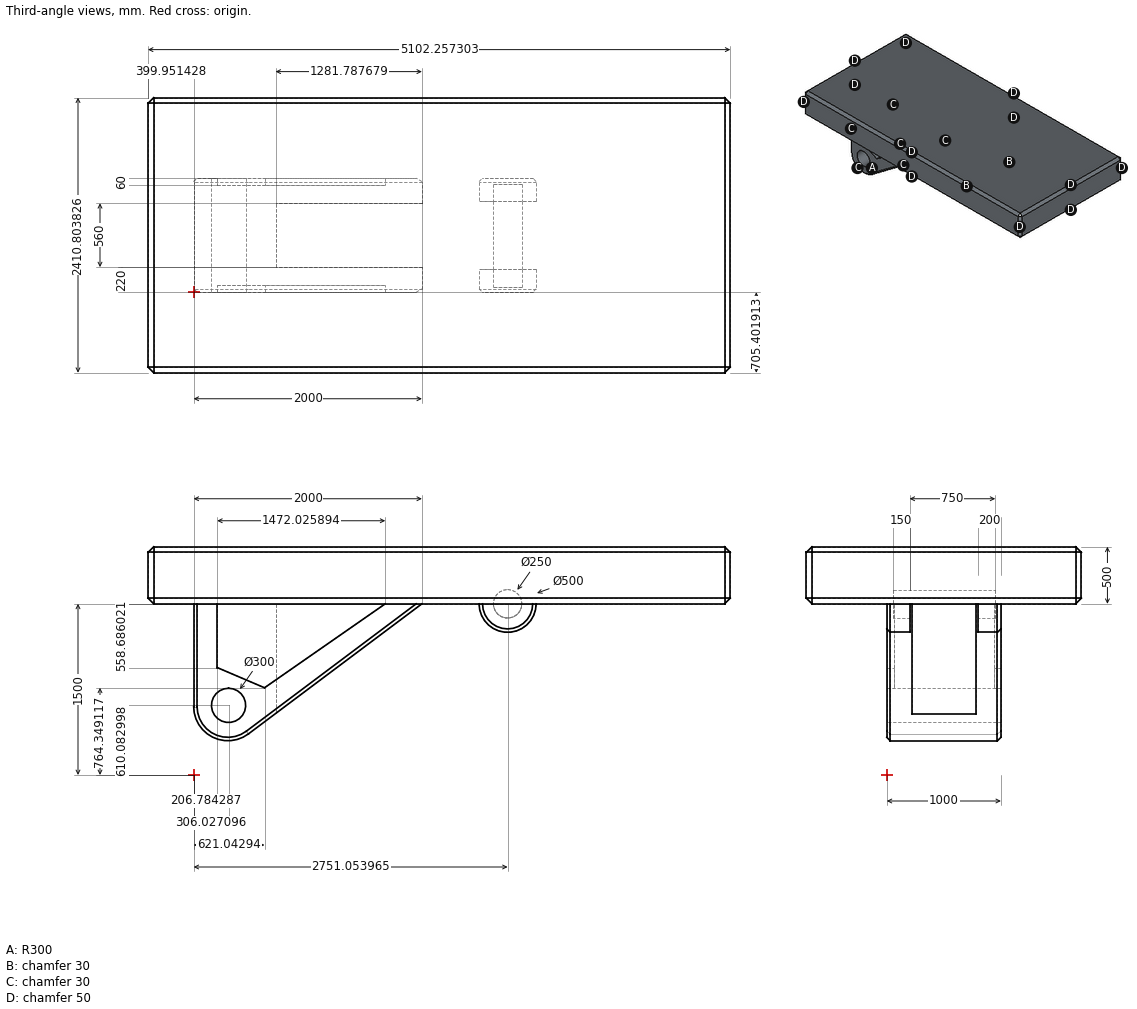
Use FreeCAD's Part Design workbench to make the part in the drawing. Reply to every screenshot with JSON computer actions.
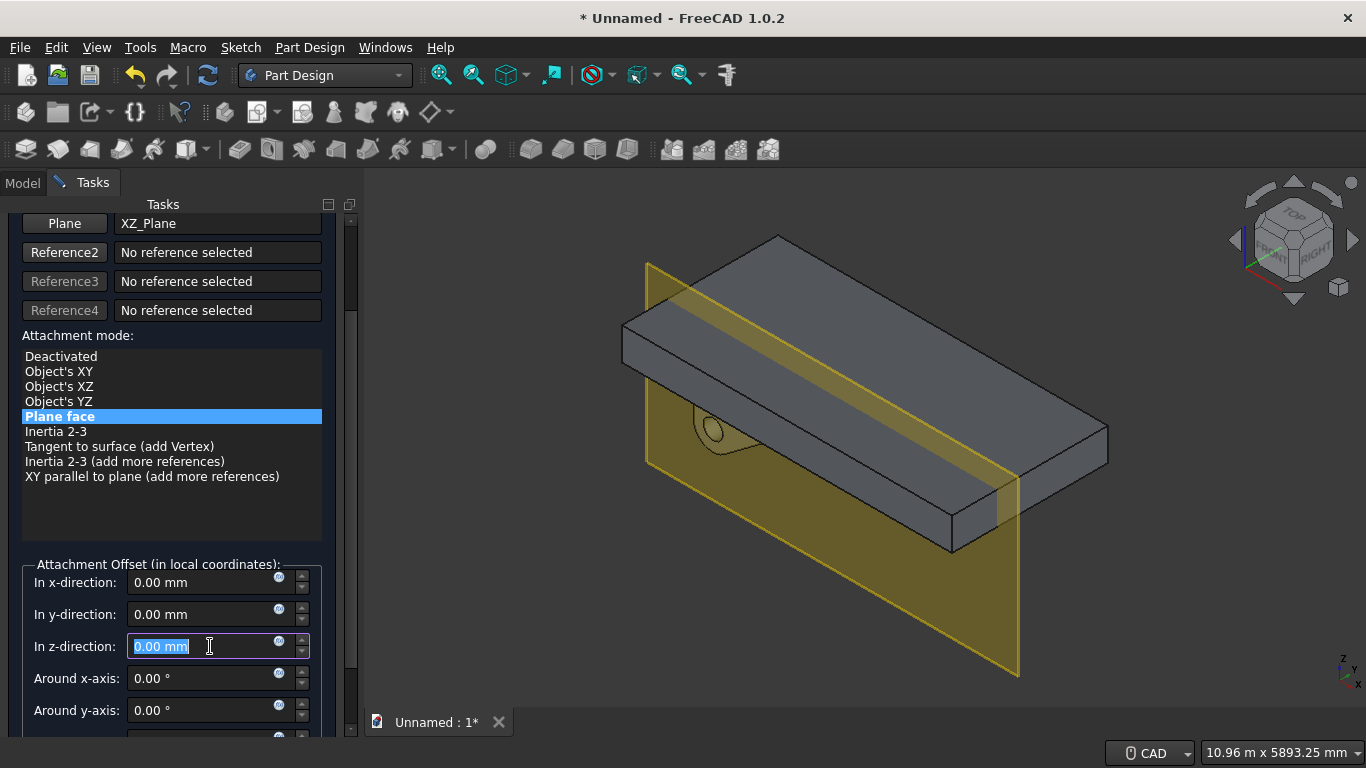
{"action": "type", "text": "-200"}
{"action": "key", "text": "Tab"}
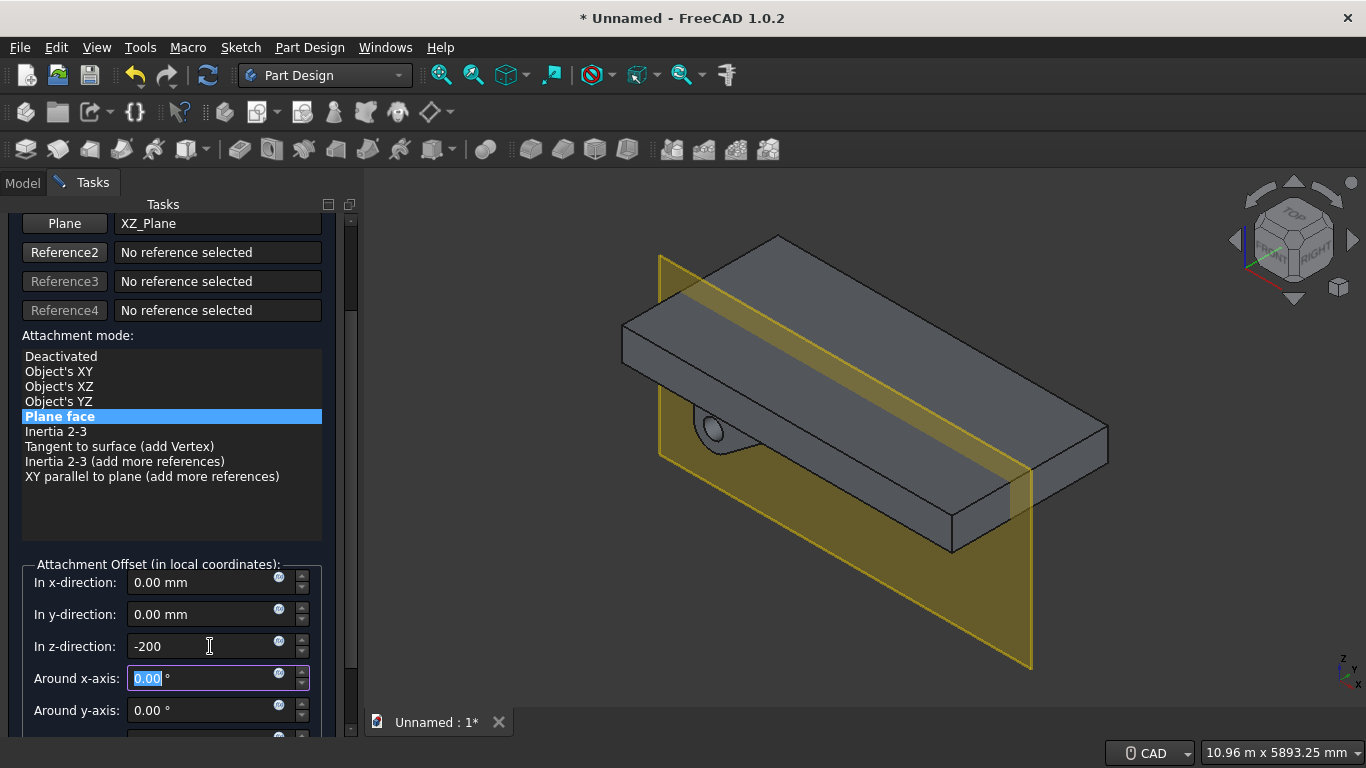
{"action": "scroll", "coordinate": [351, 475], "scroll_direction": "up", "scroll_amount": 3}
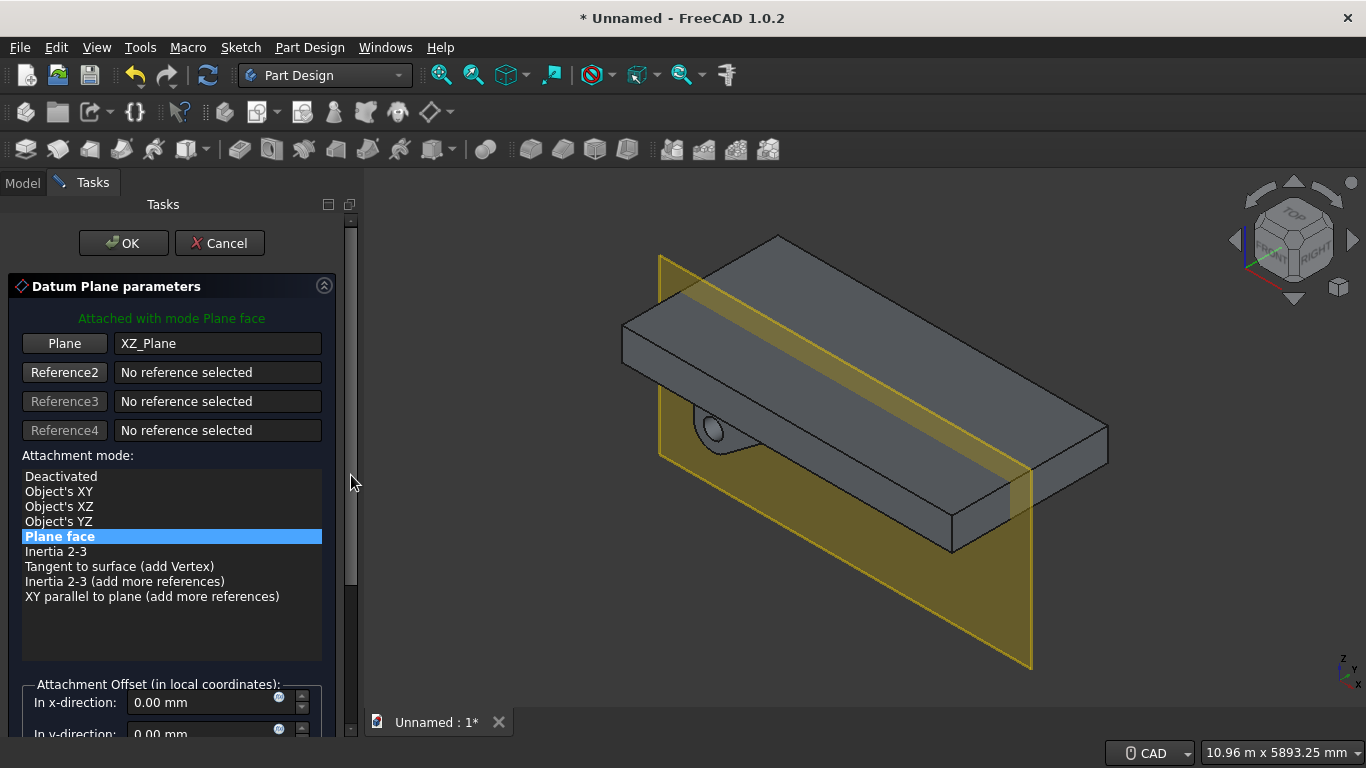
{"action": "left_click", "coordinate": [124, 243]}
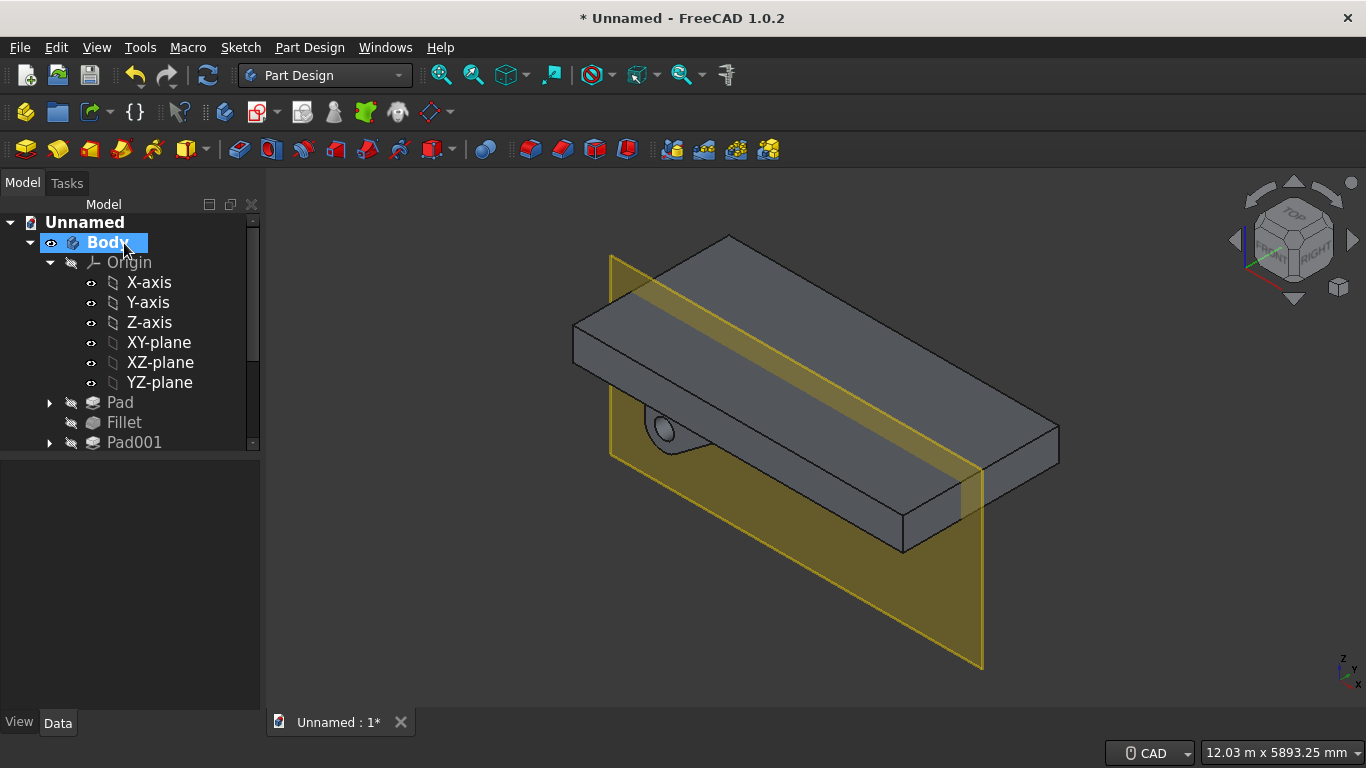
{"action": "scroll", "coordinate": [100, 338], "scroll_direction": "down", "scroll_amount": 3}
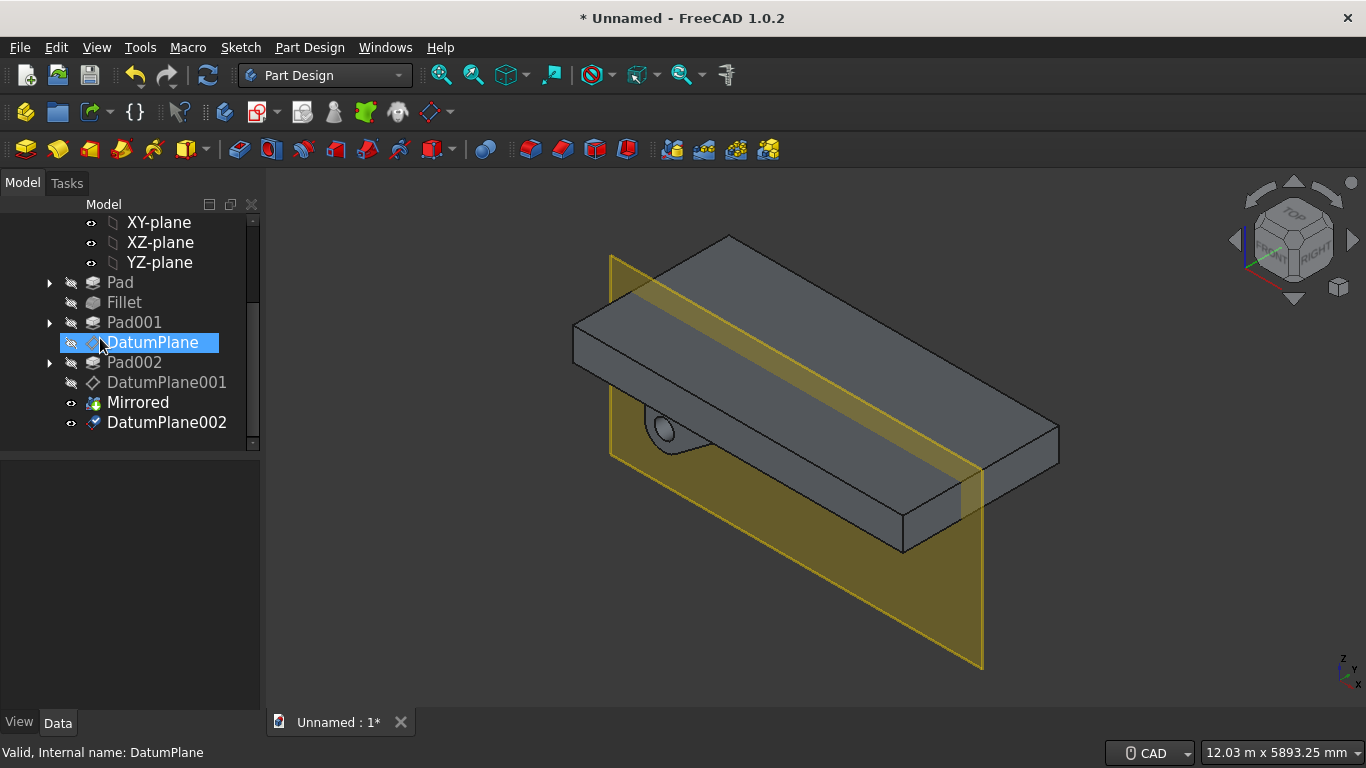
{"action": "left_click", "coordinate": [116, 423]}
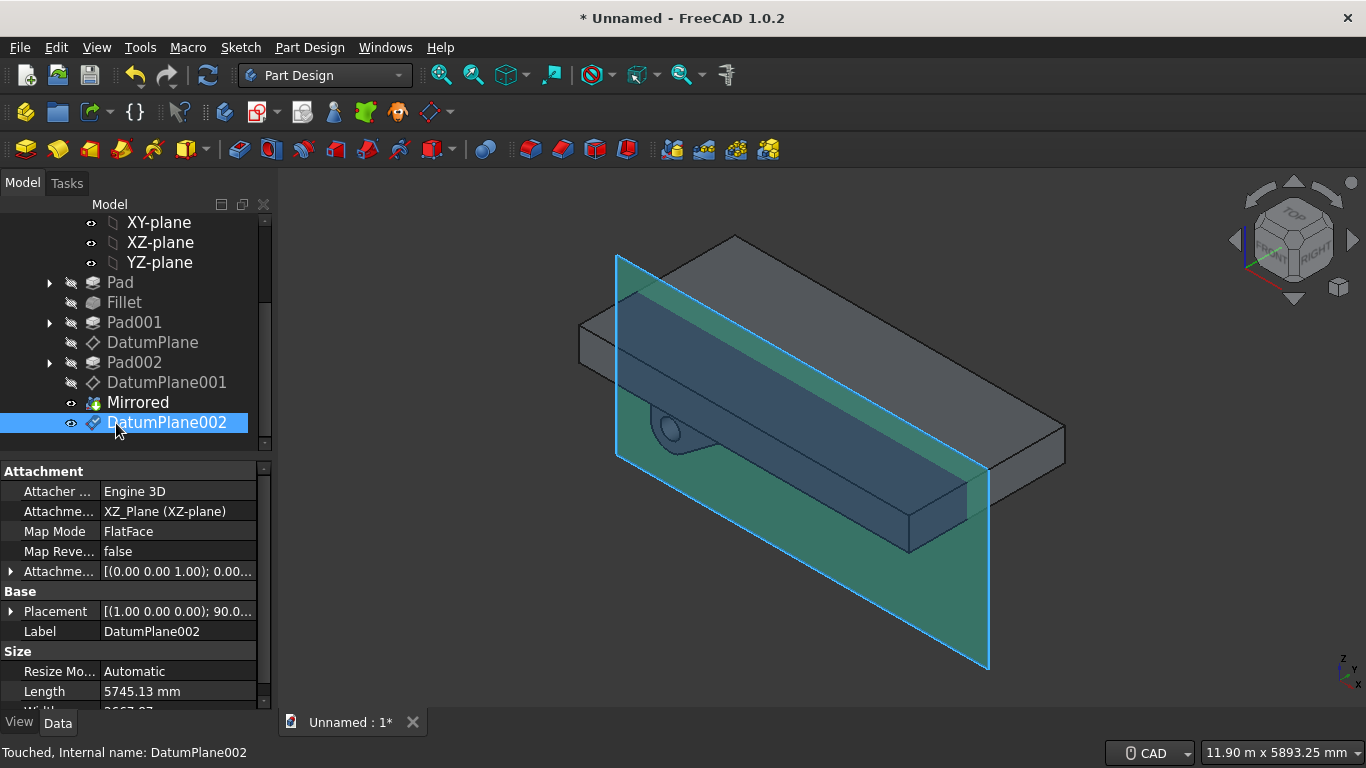
{"action": "left_click", "coordinate": [258, 112]}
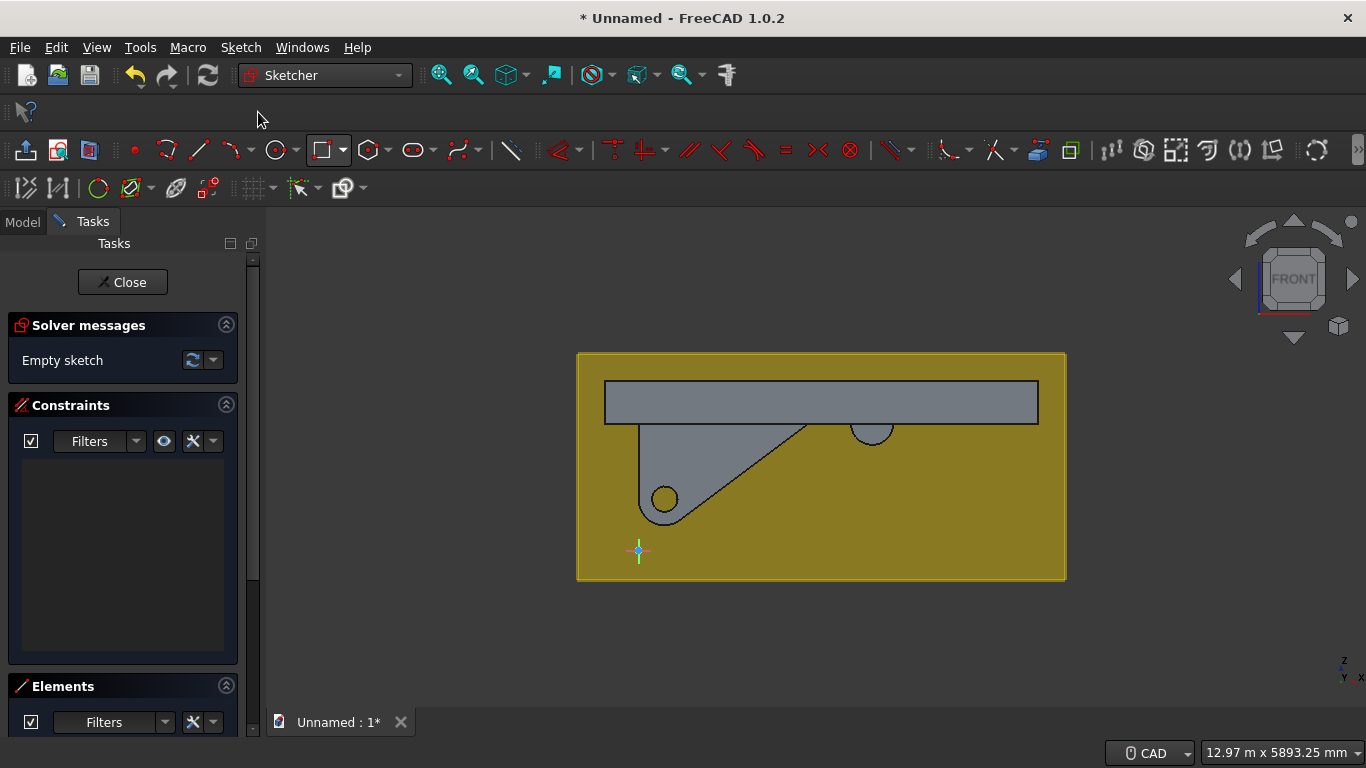
{"action": "key", "text": "q s"}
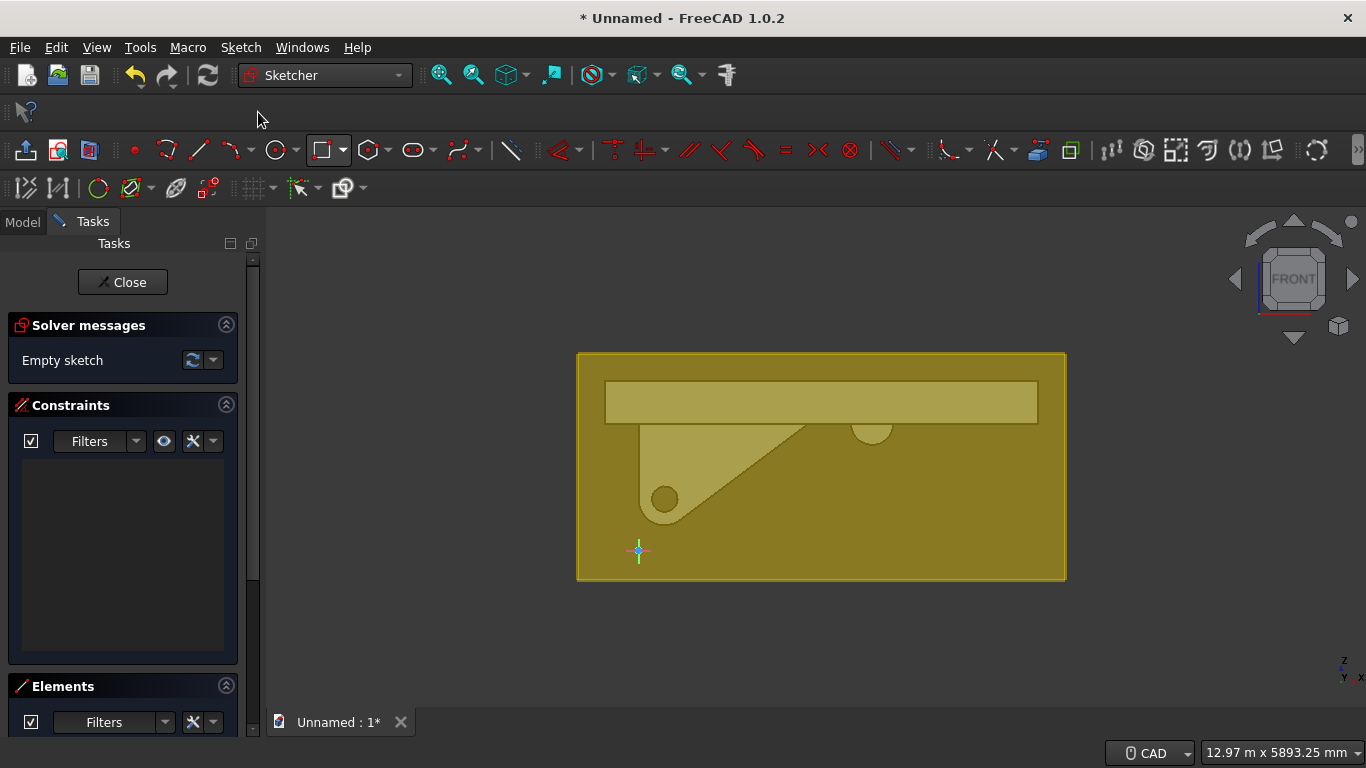
{"action": "scroll", "coordinate": [882, 421], "scroll_direction": "up", "scroll_amount": 13}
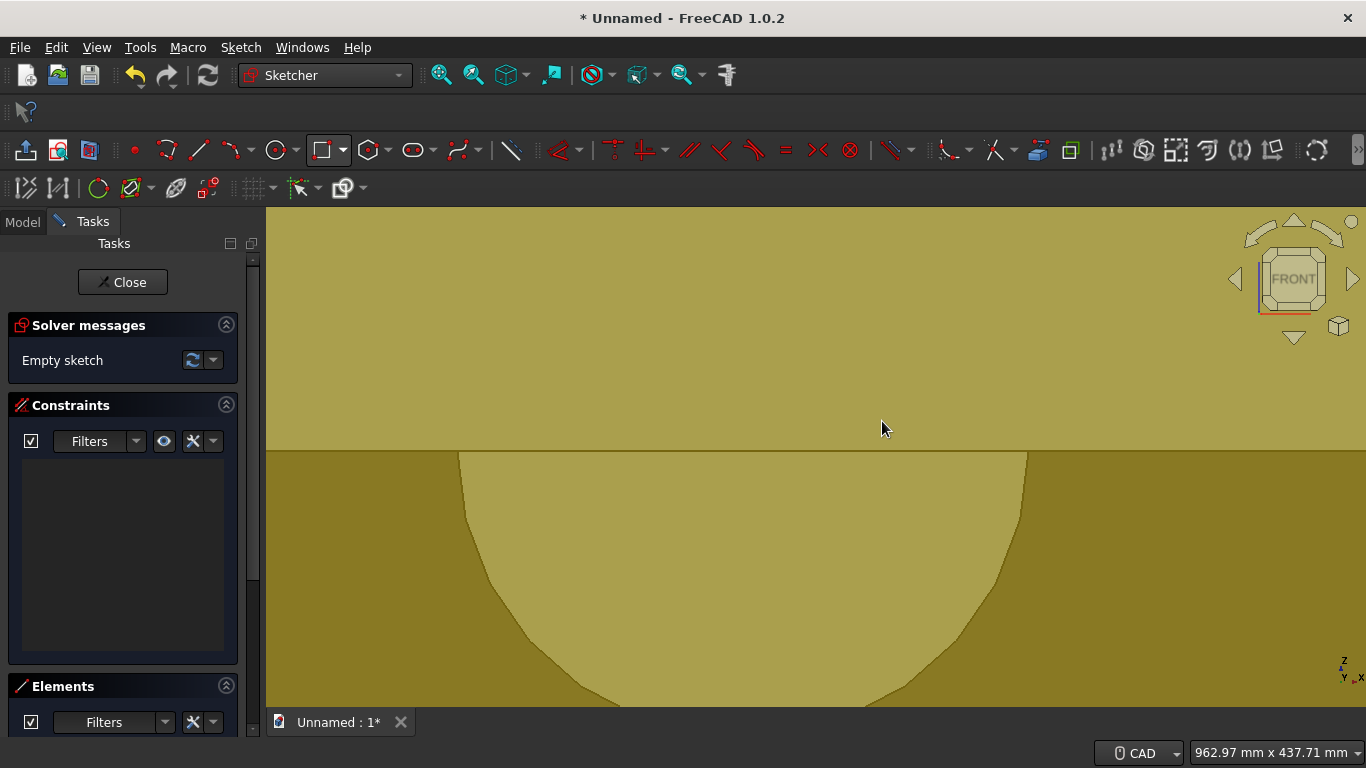
{"action": "left_click", "coordinate": [276, 150]}